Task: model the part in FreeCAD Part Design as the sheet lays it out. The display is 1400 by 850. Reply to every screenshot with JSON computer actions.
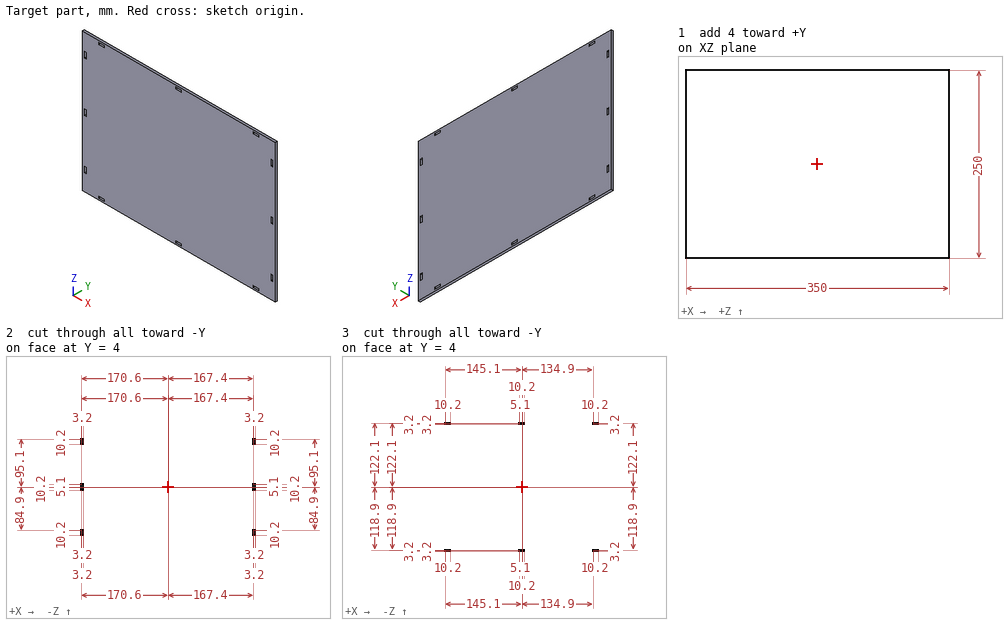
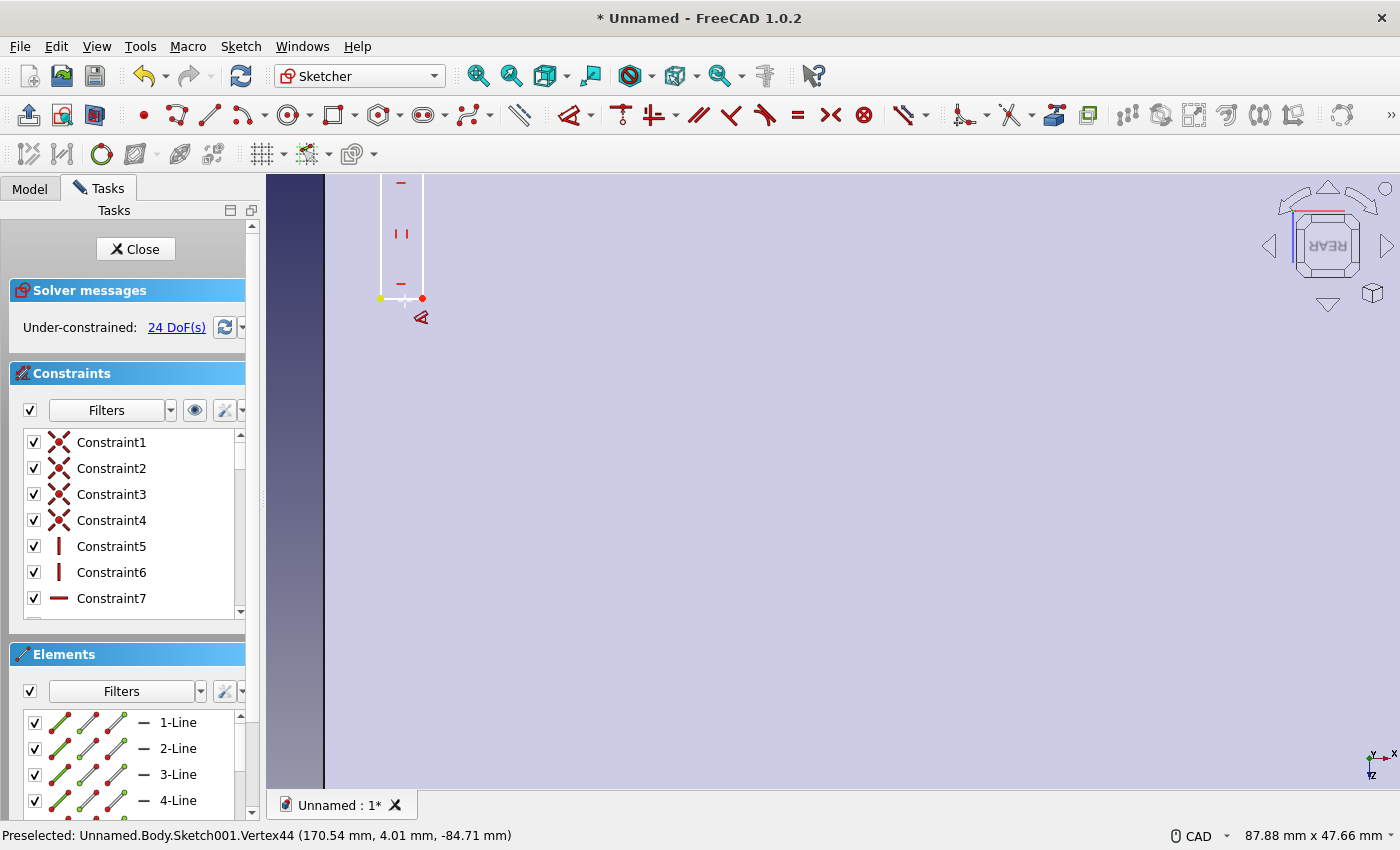
{"action": "left_click", "coordinate": [402, 299]}
{"action": "left_click", "coordinate": [402, 265]}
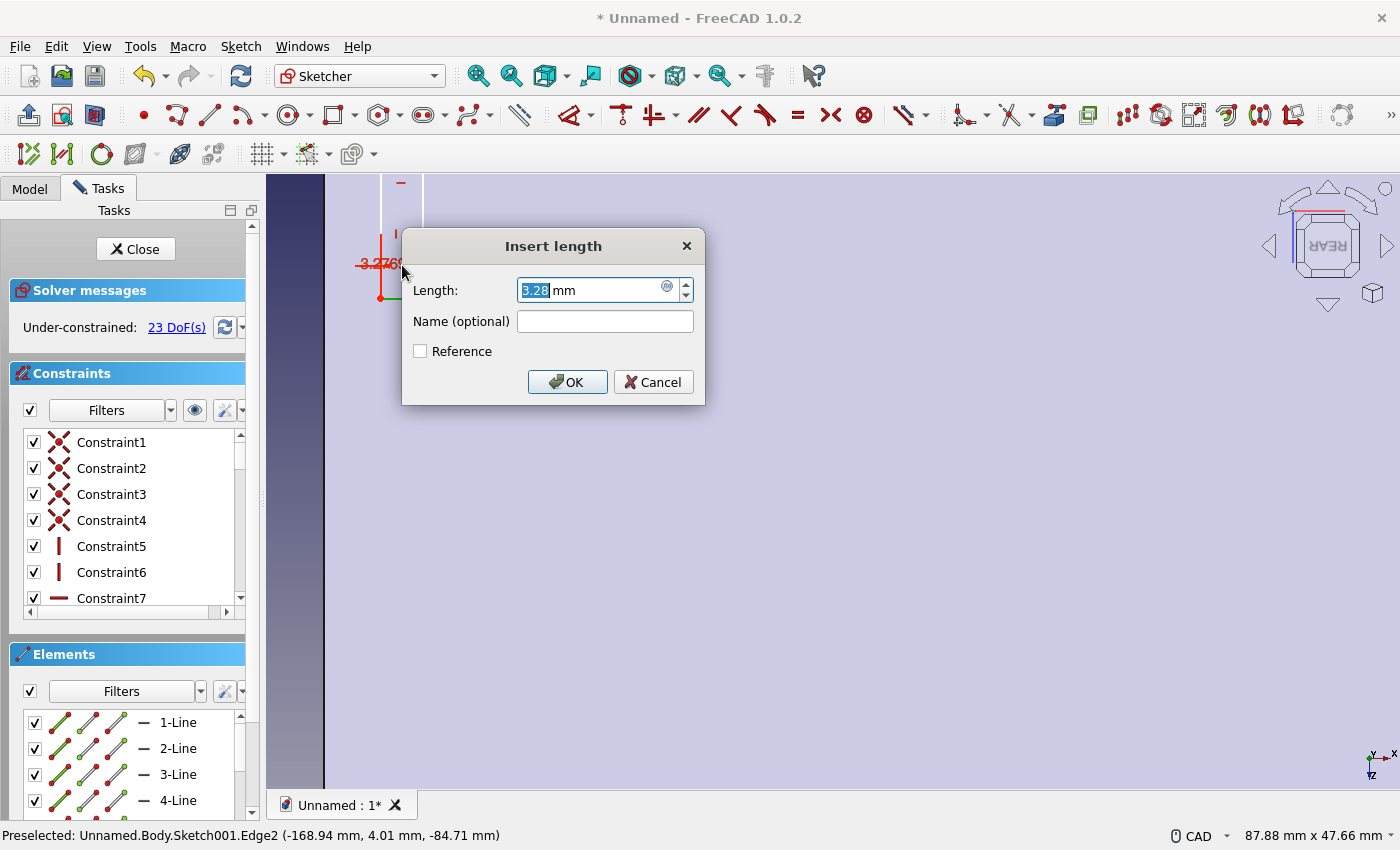
{"action": "type", "text": "3.2"}
{"action": "key", "text": "Return"}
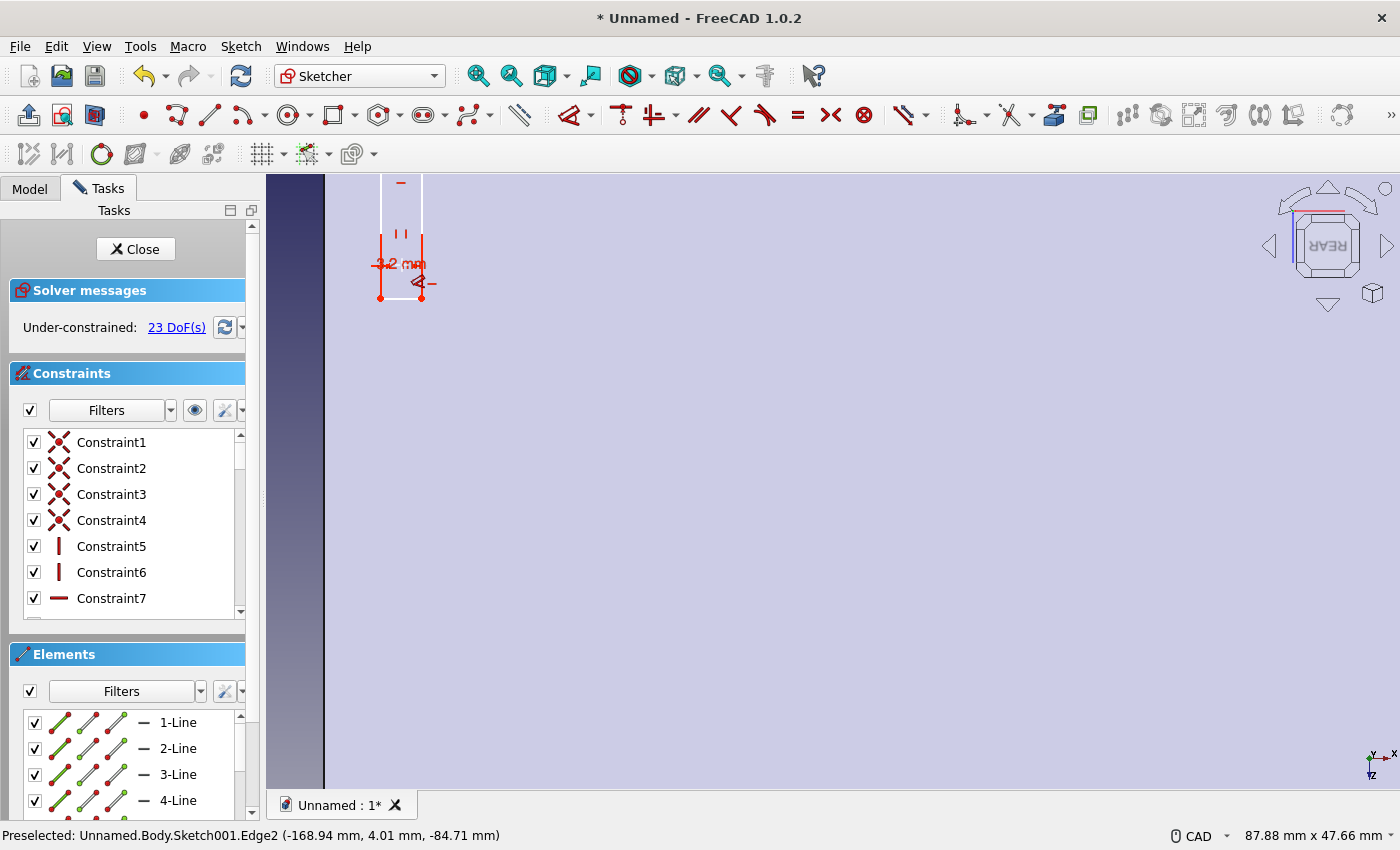
{"action": "scroll", "coordinate": [405, 301], "scroll_direction": "down", "scroll_amount": 9}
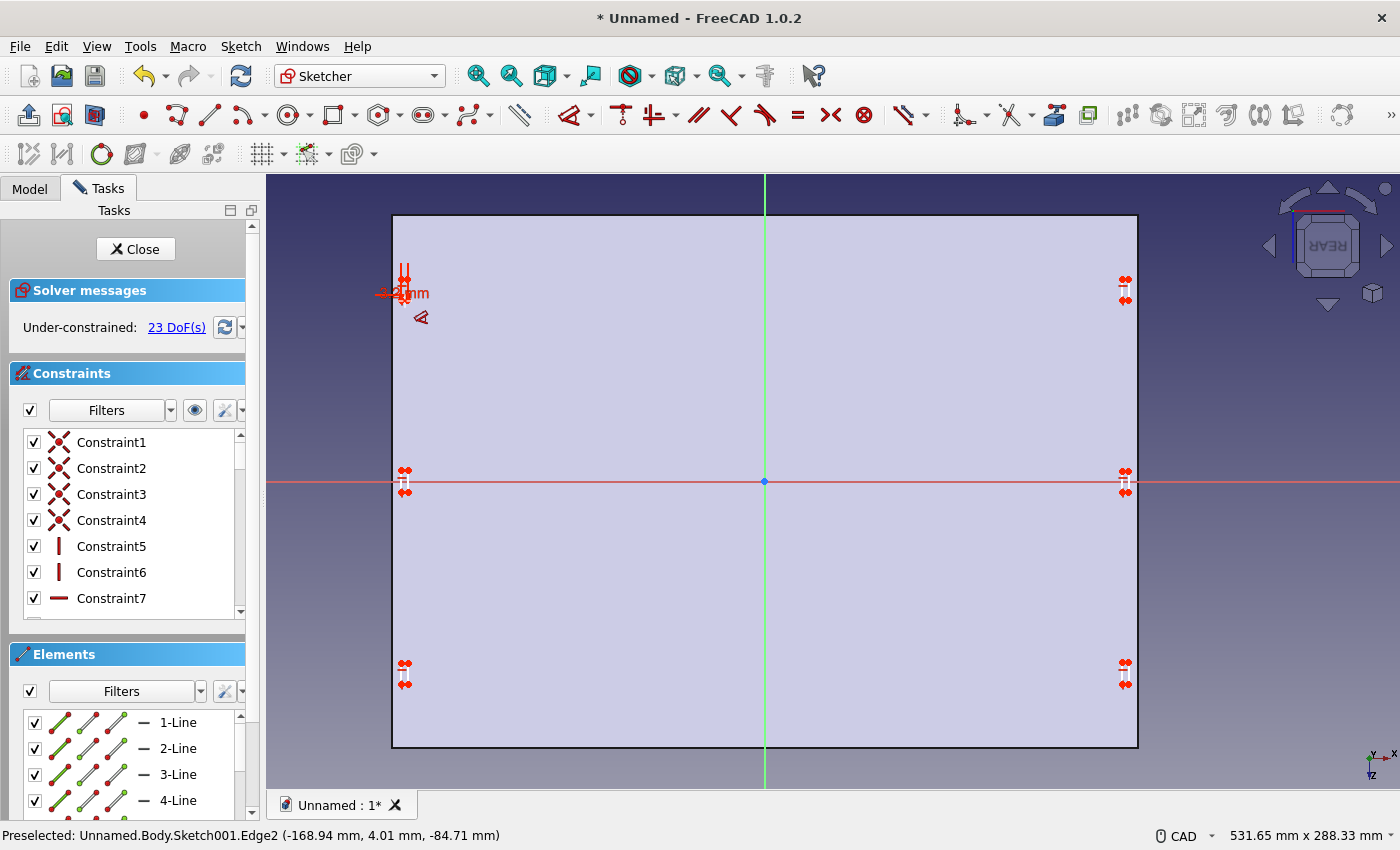
{"action": "scroll", "coordinate": [403, 493], "scroll_direction": "up", "scroll_amount": 10}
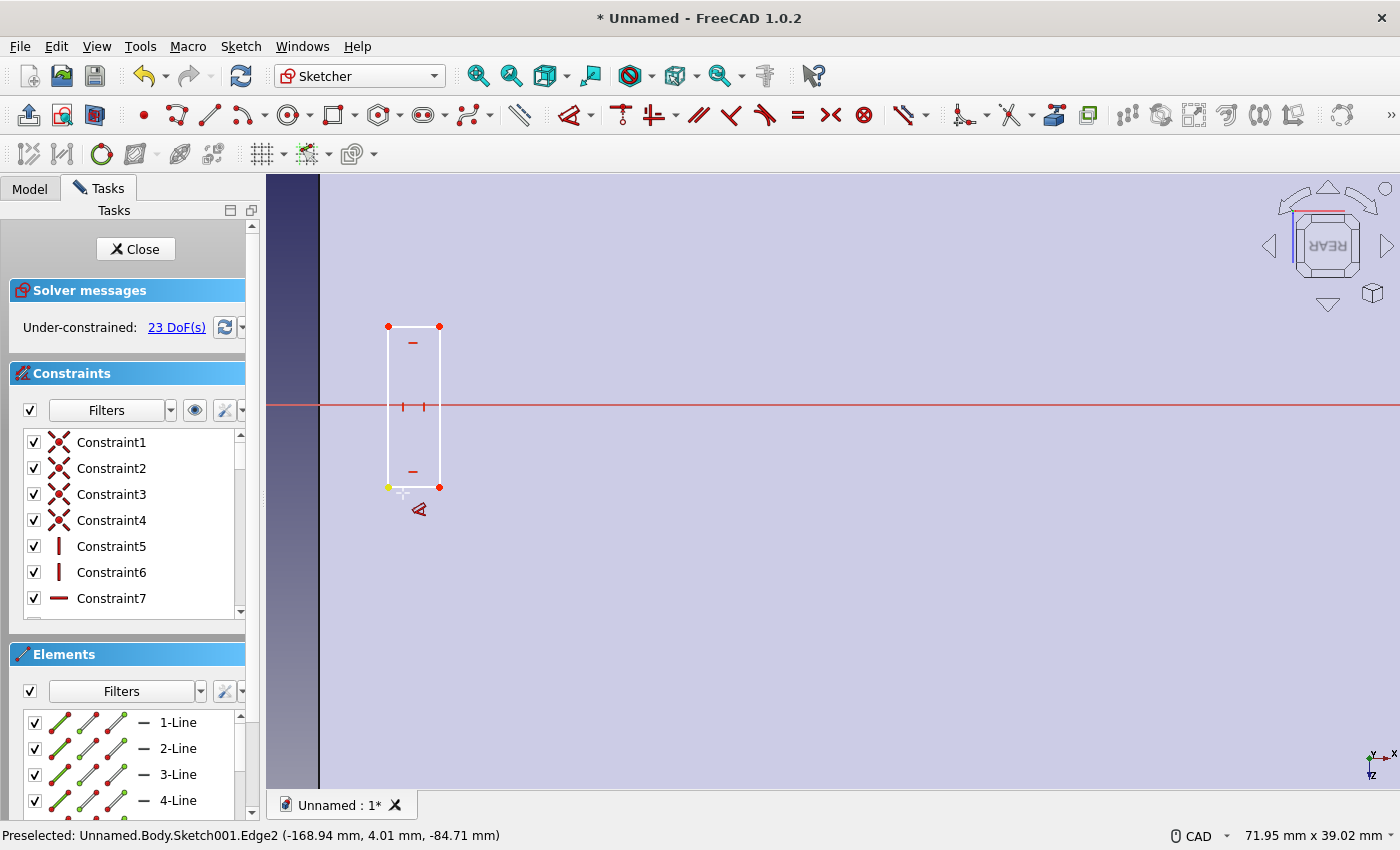
{"action": "left_click", "coordinate": [404, 487]}
{"action": "left_click", "coordinate": [414, 521]}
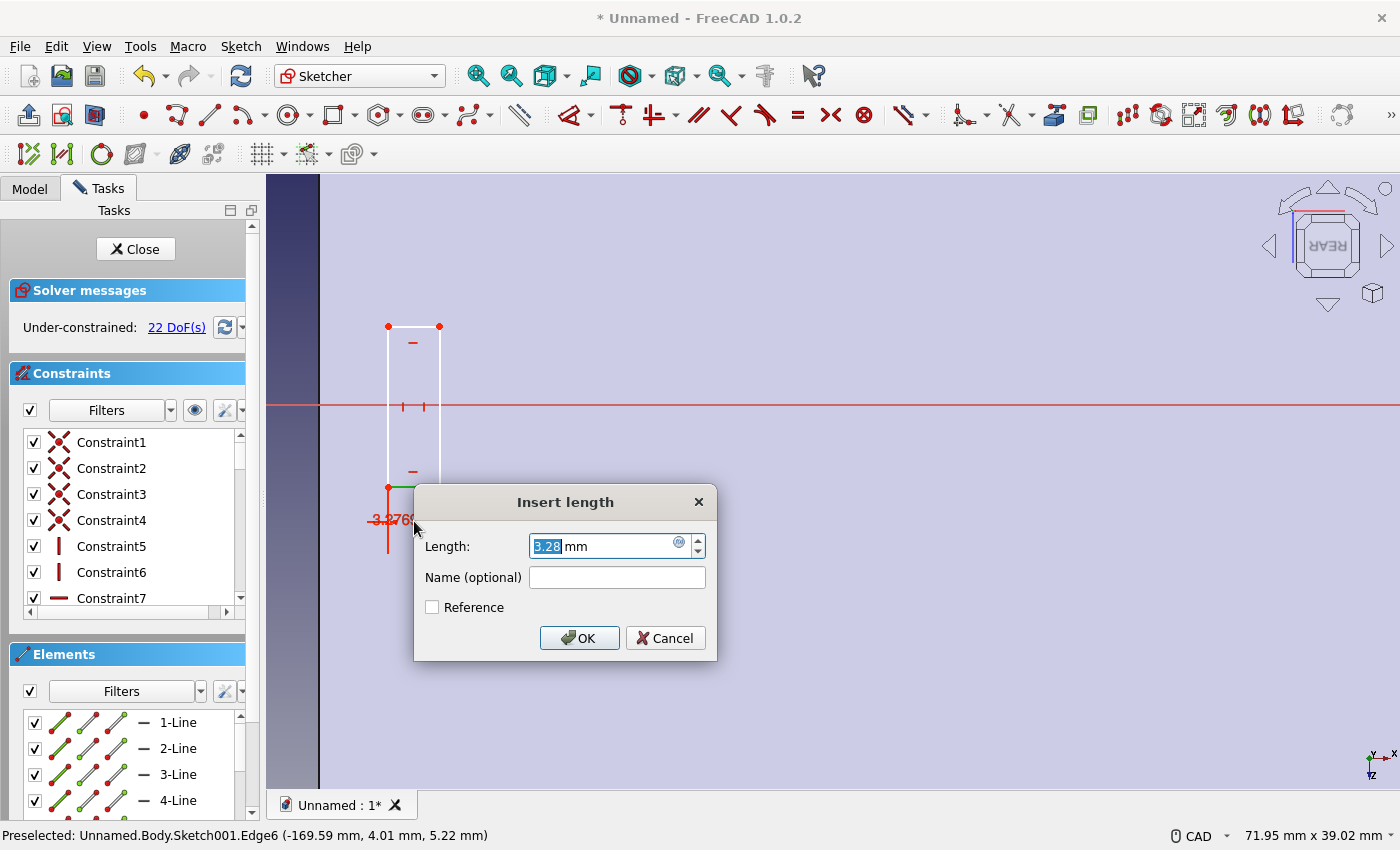
{"action": "type", "text": "3.2"}
{"action": "key", "text": "Return"}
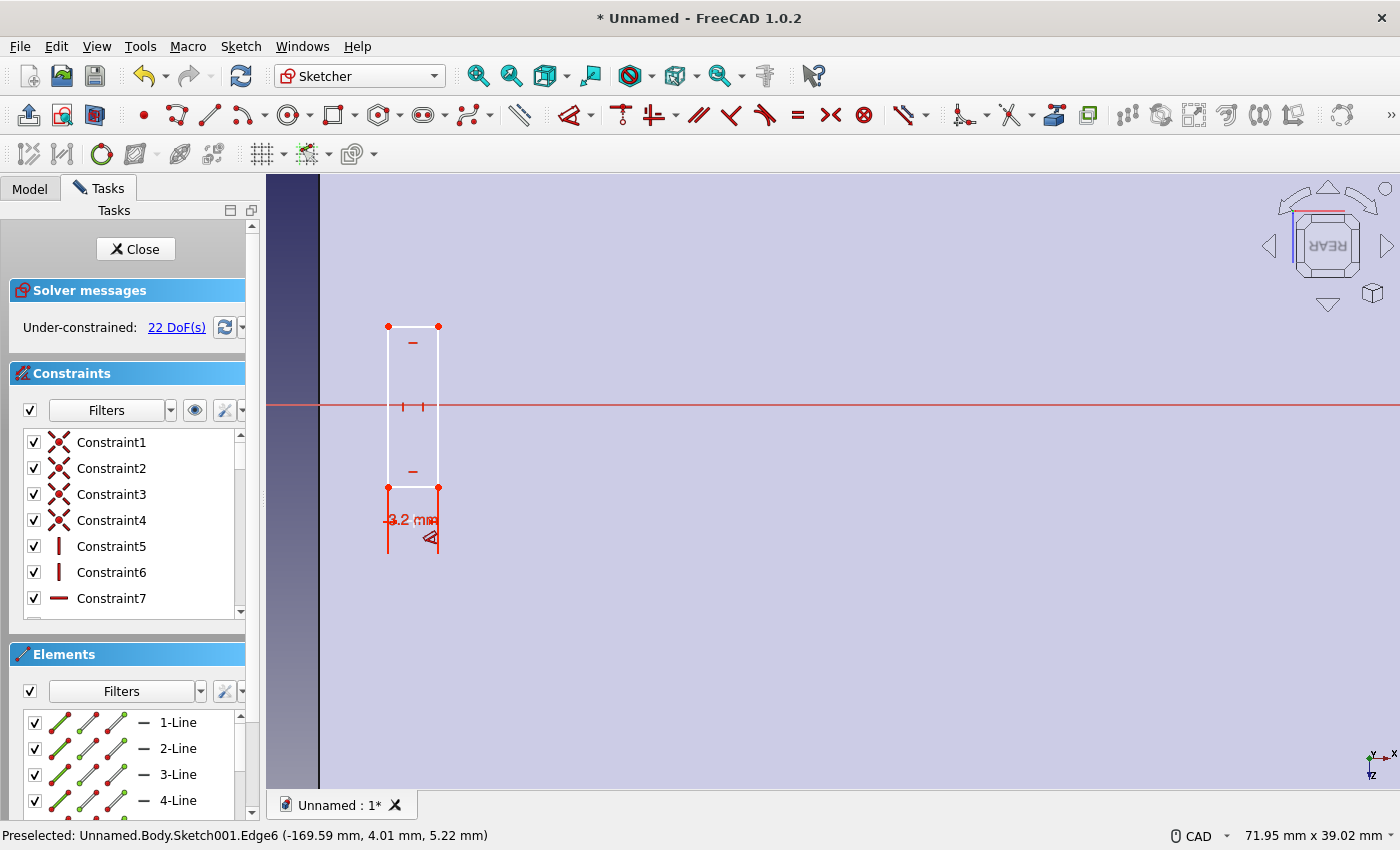
{"action": "scroll", "coordinate": [403, 494], "scroll_direction": "down", "scroll_amount": 10}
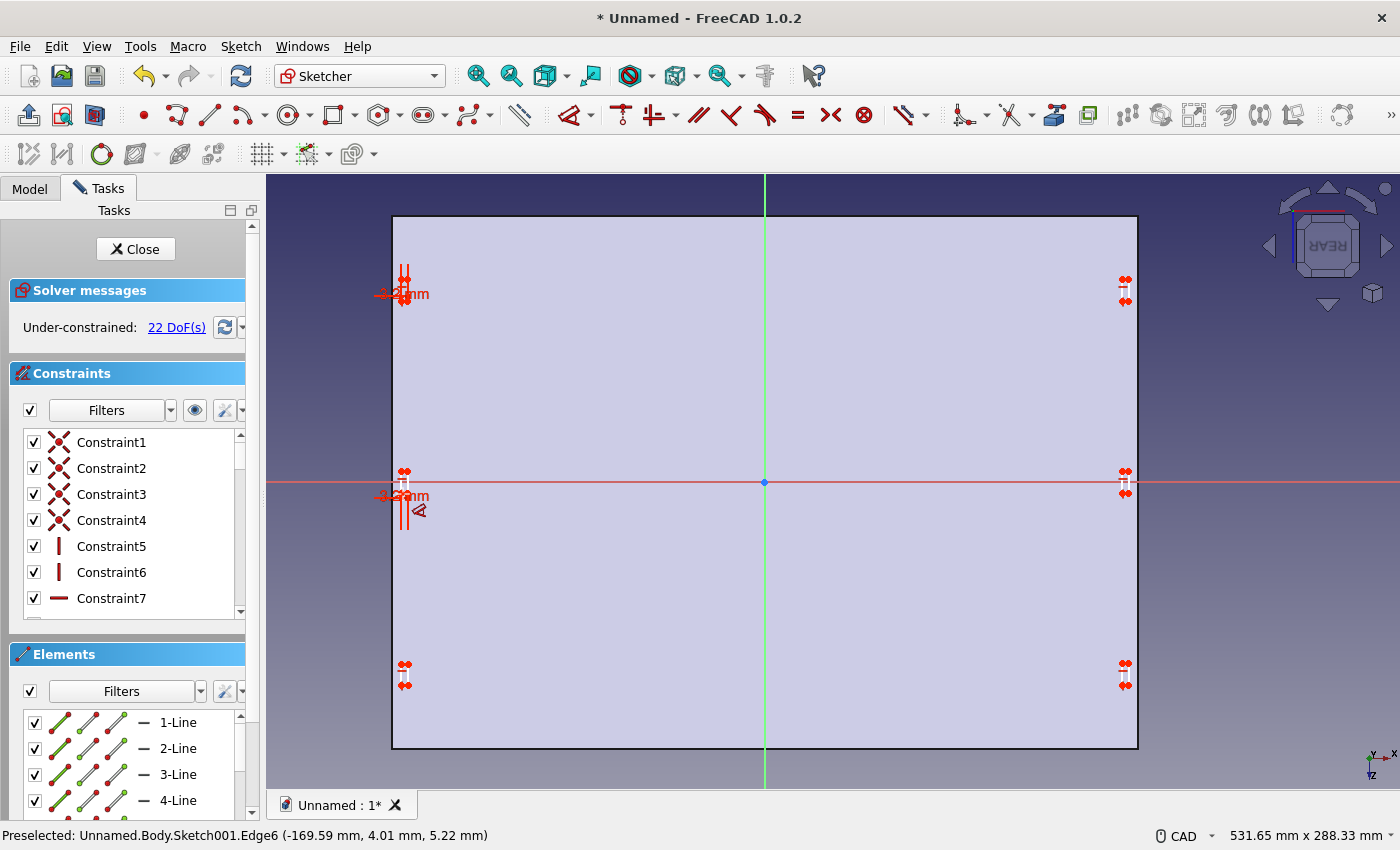
{"action": "scroll", "coordinate": [403, 686], "scroll_direction": "up", "scroll_amount": 10}